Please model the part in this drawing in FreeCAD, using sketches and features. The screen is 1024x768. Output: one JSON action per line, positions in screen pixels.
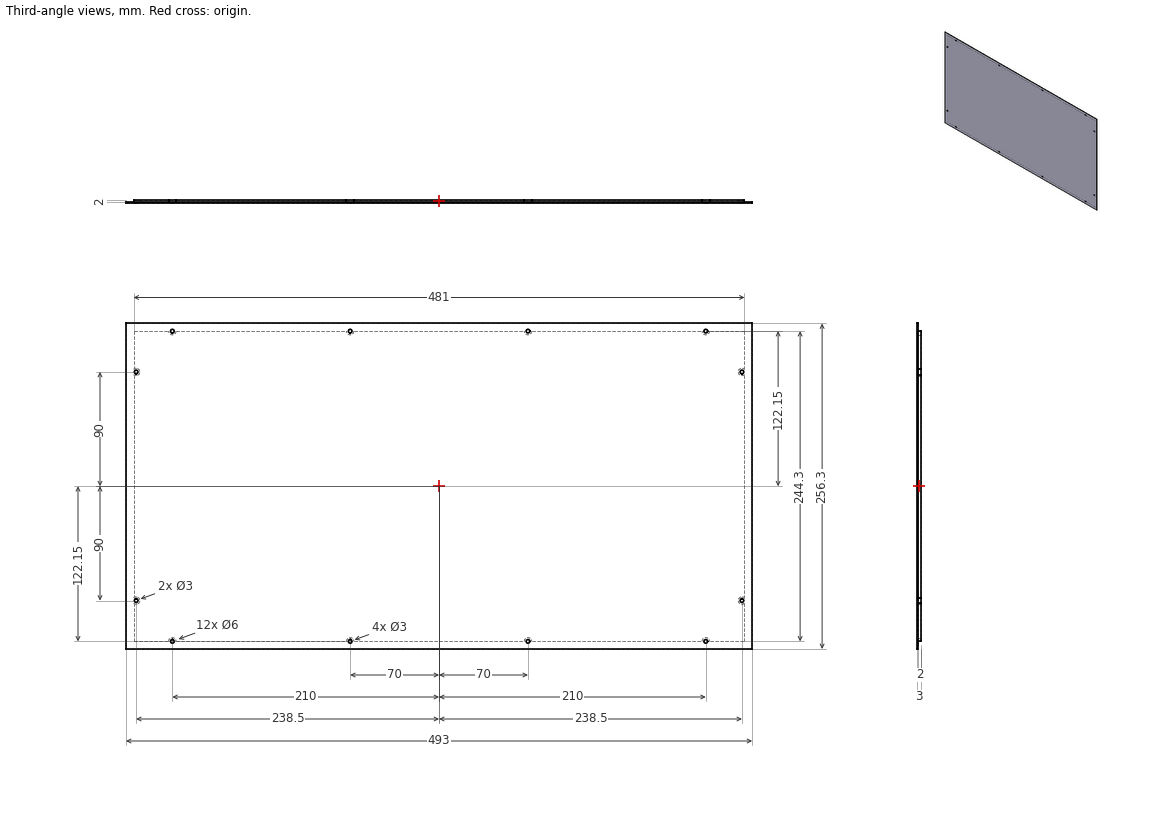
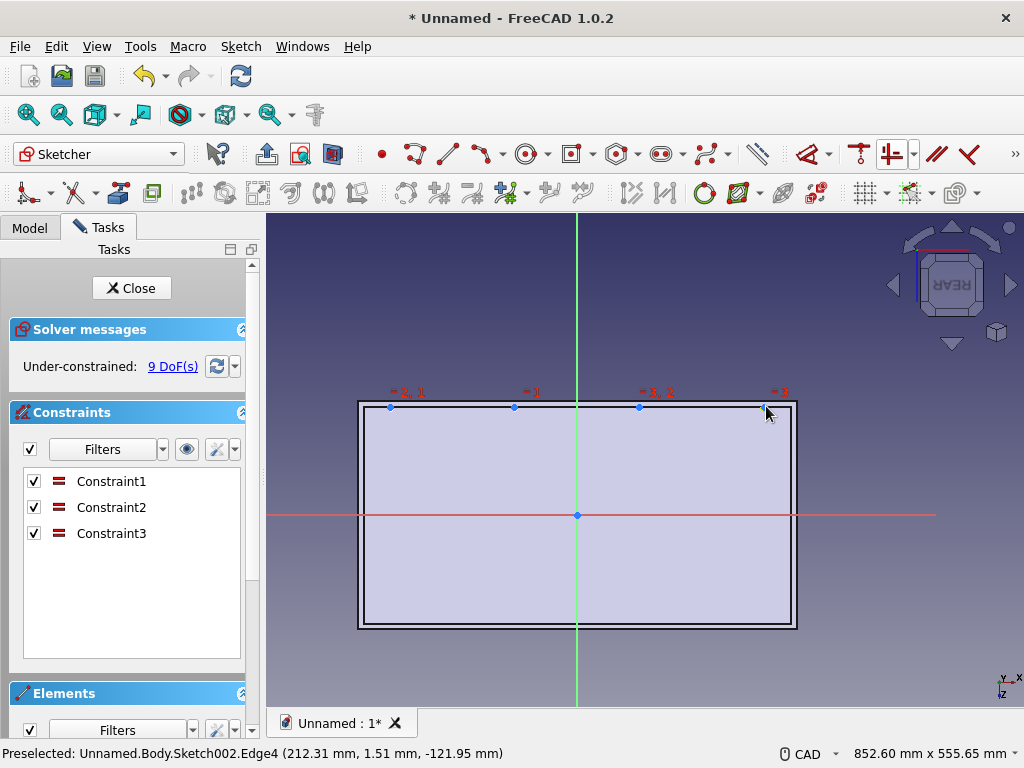
{"action": "left_click", "coordinate": [515, 408]}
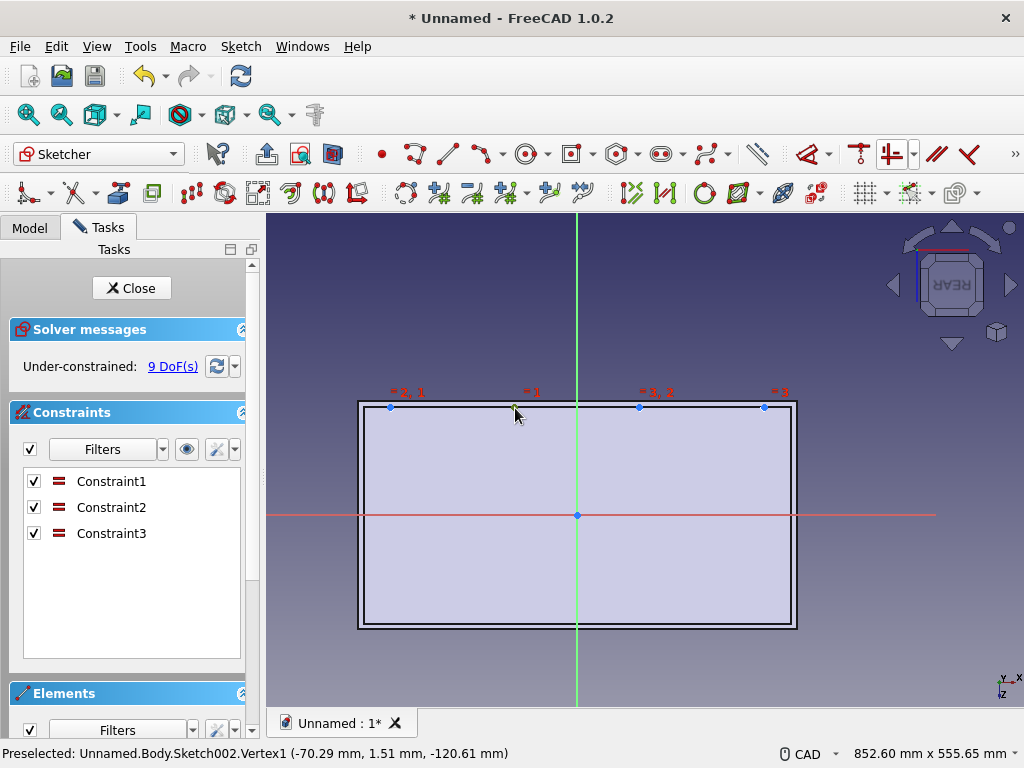
{"action": "left_click", "coordinate": [391, 408]}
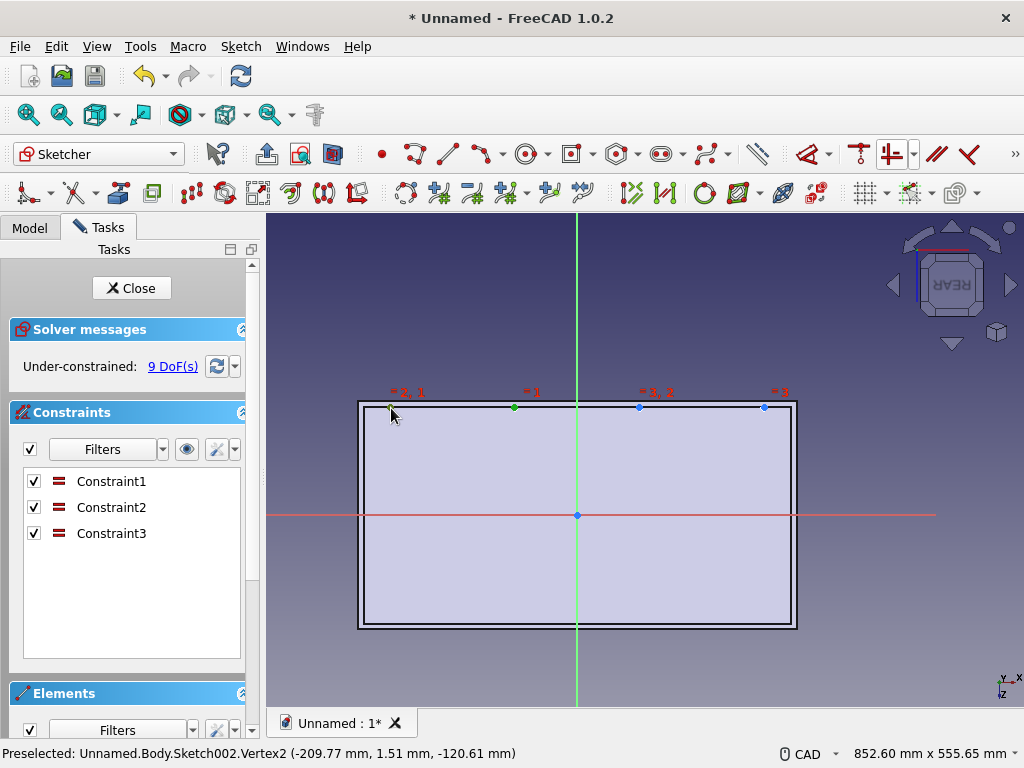
{"action": "left_click", "coordinate": [914, 154]}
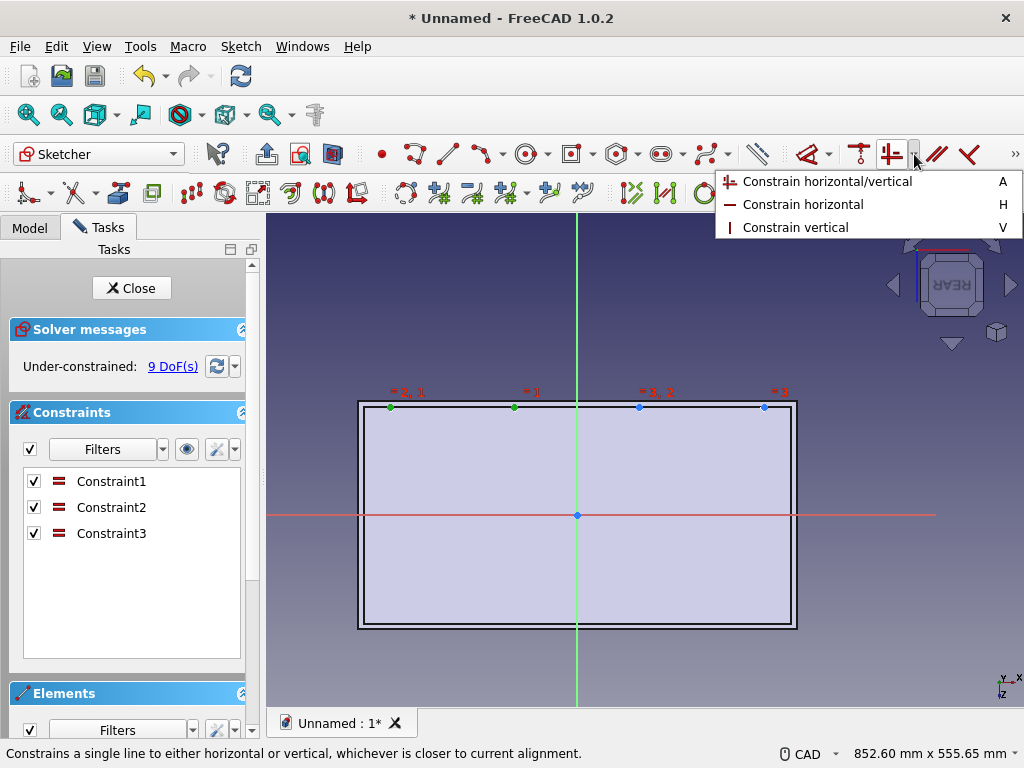
{"action": "left_click", "coordinate": [869, 204]}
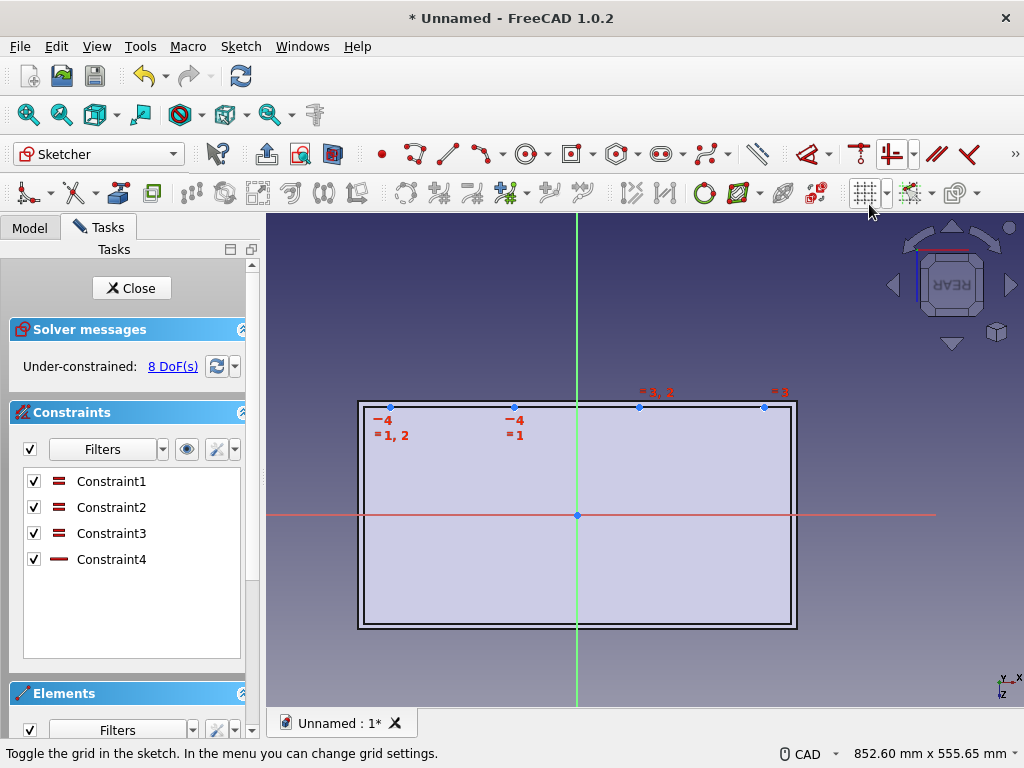
{"action": "left_click", "coordinate": [515, 408]}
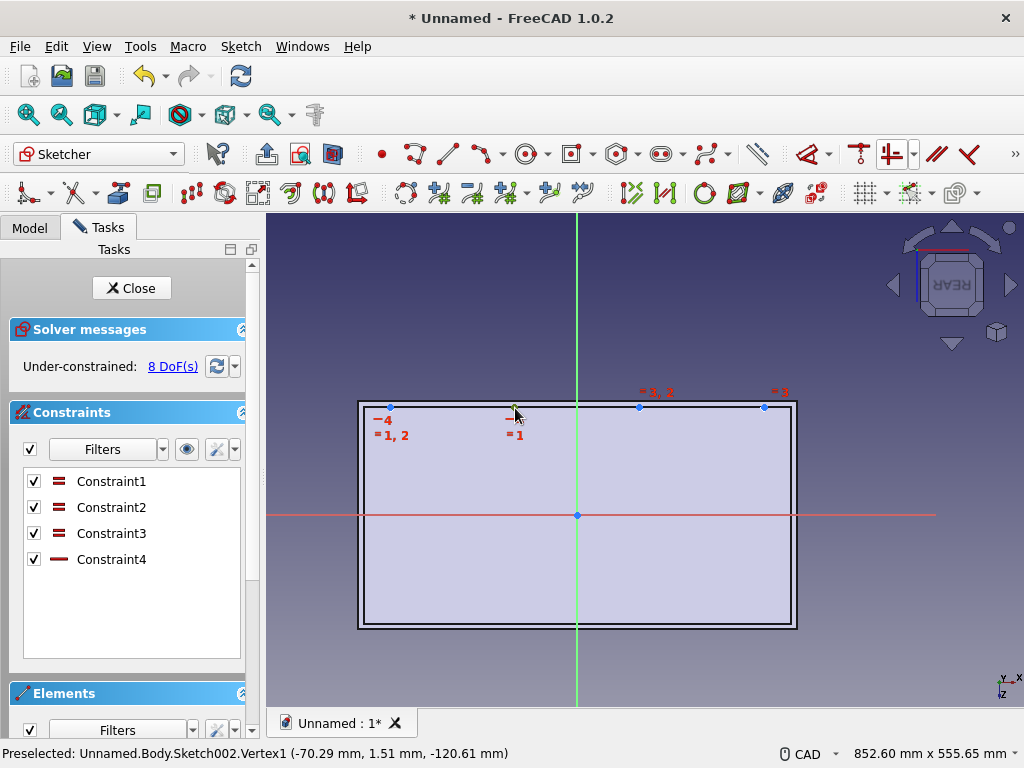
{"action": "left_click", "coordinate": [640, 408]}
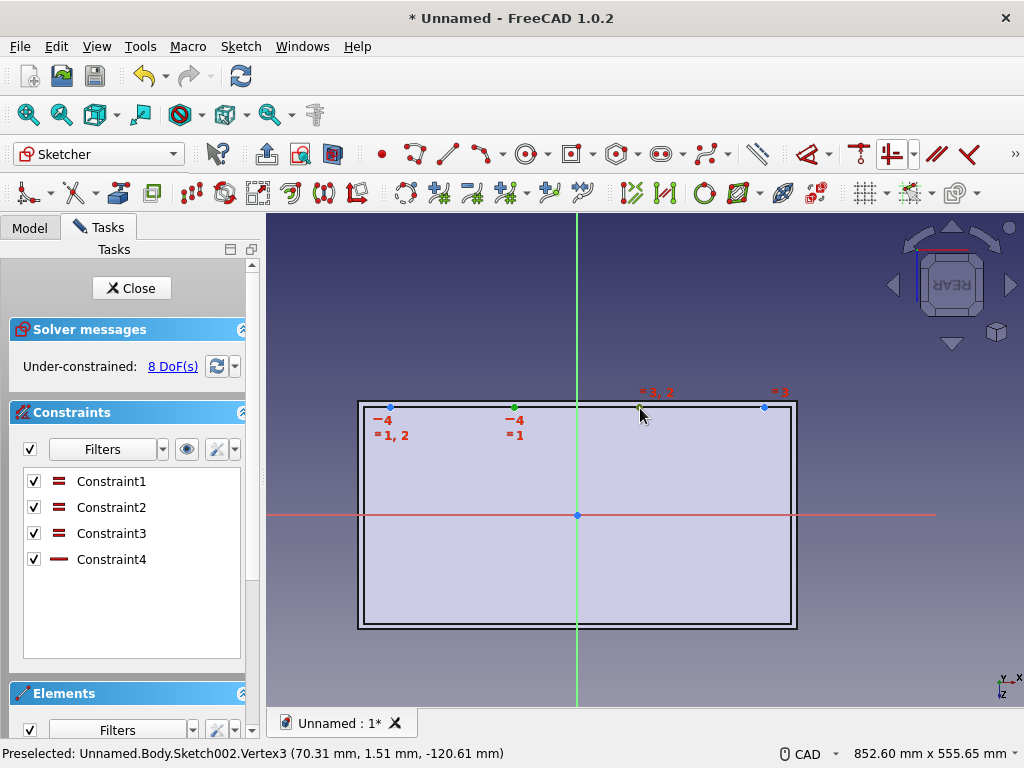
{"action": "left_click", "coordinate": [914, 154]}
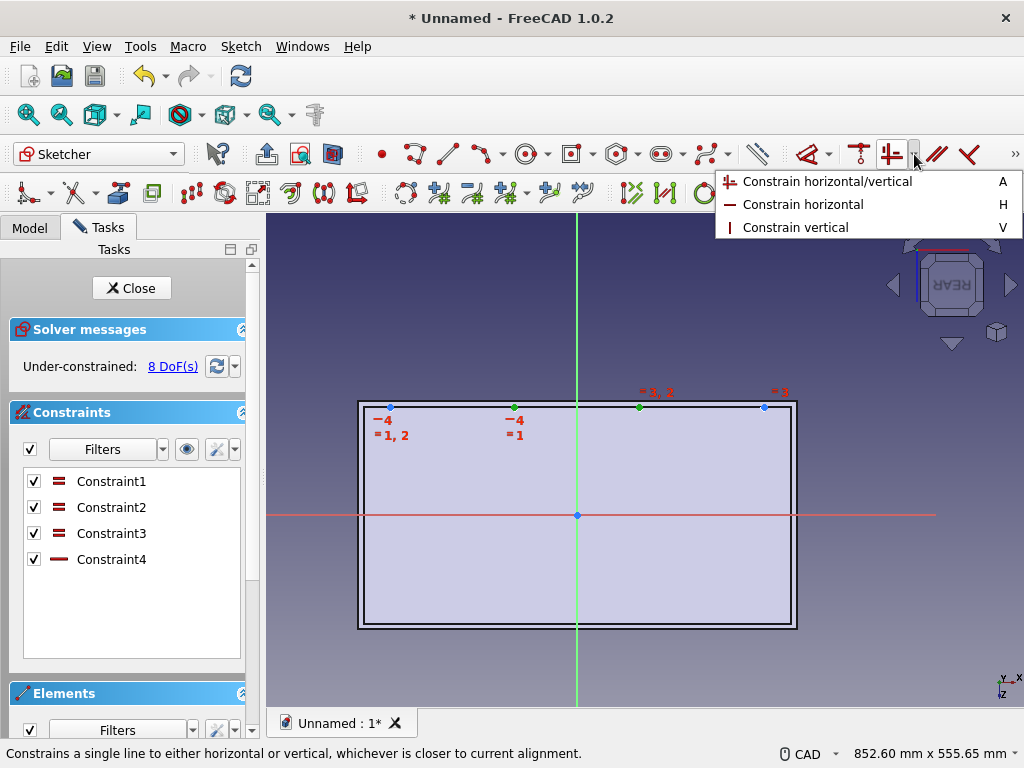
{"action": "left_click", "coordinate": [869, 204]}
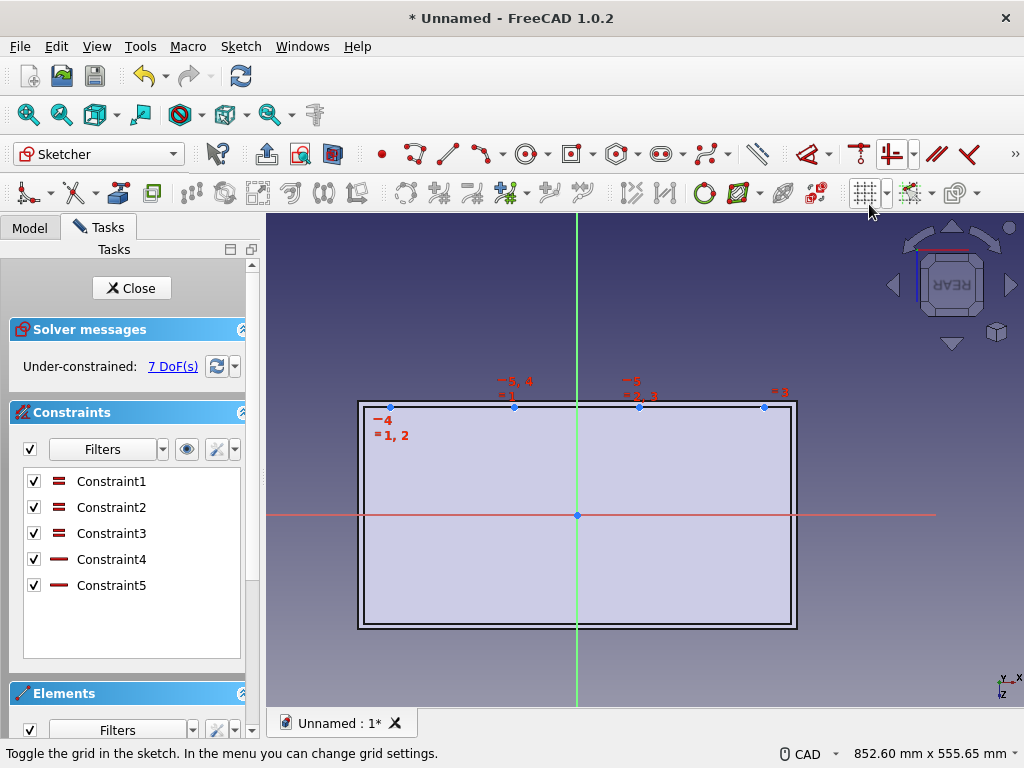
{"action": "left_click", "coordinate": [640, 408]}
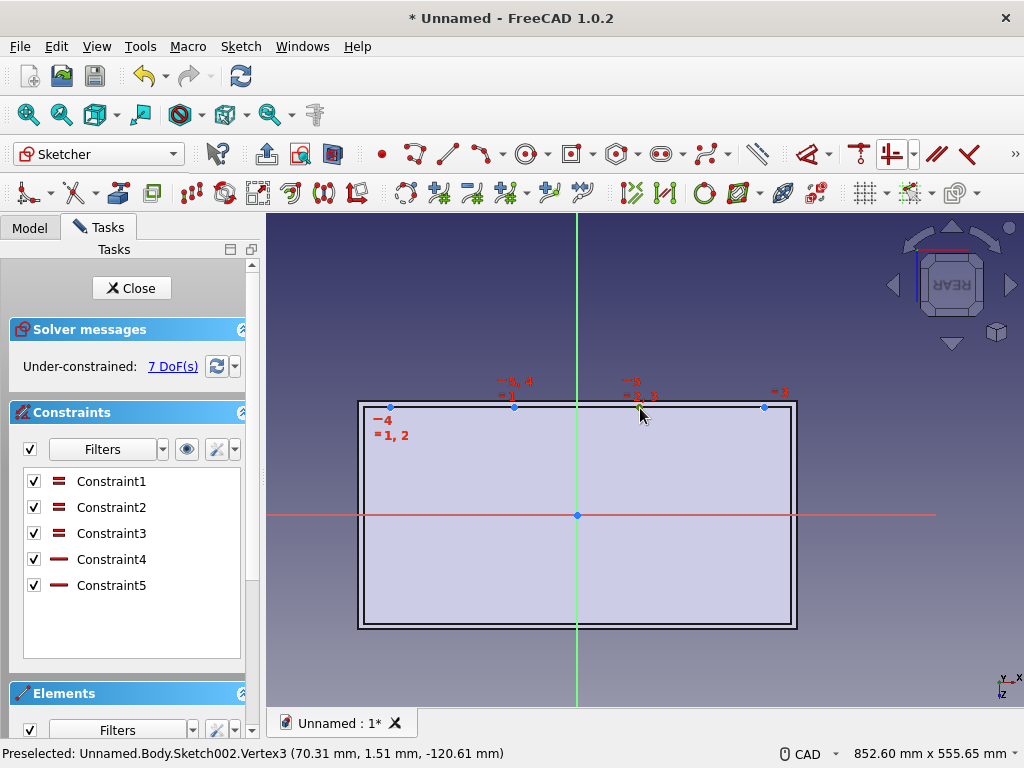
{"action": "left_click", "coordinate": [764, 408]}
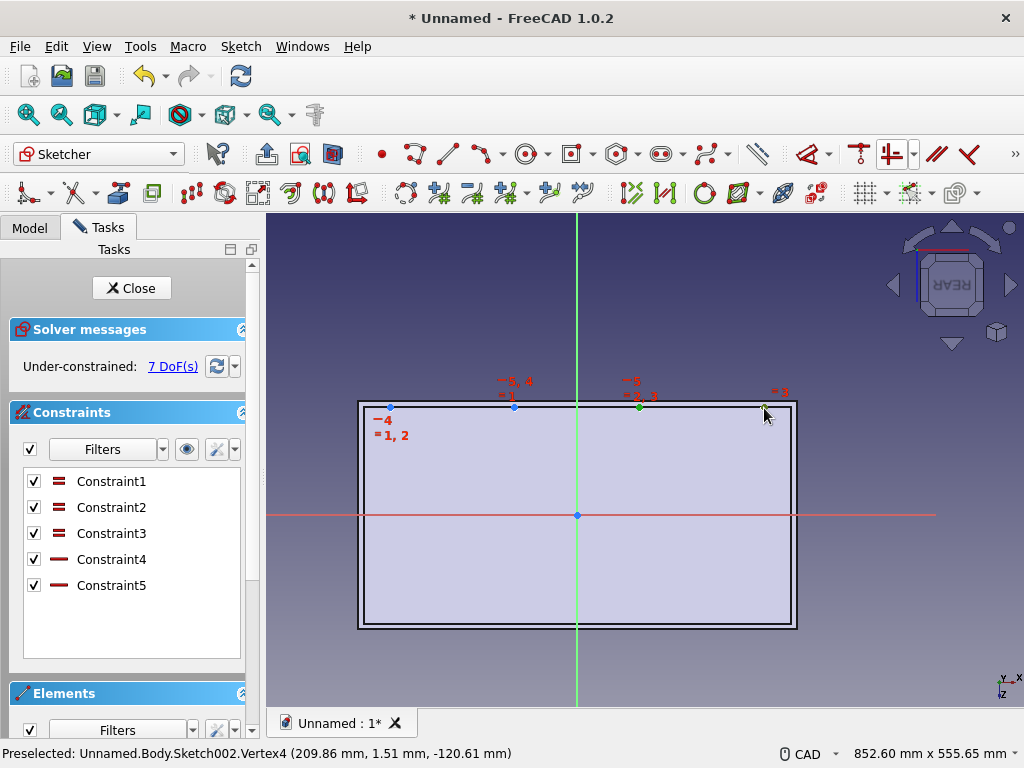
{"action": "left_click", "coordinate": [914, 154]}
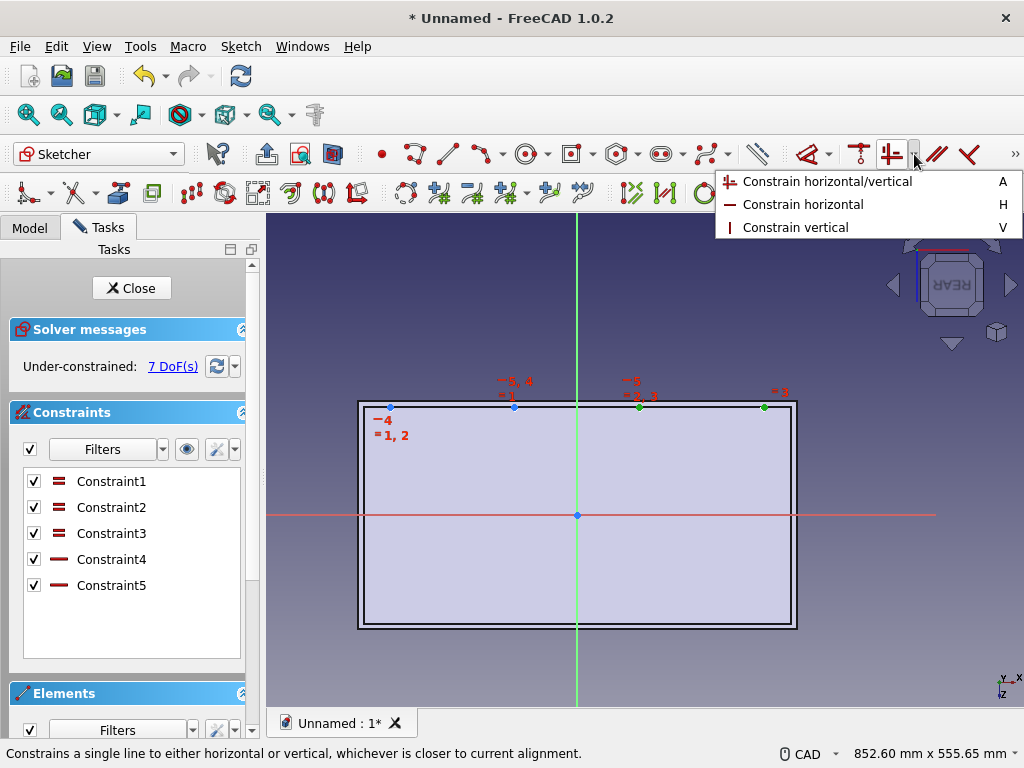
{"action": "left_click", "coordinate": [869, 204]}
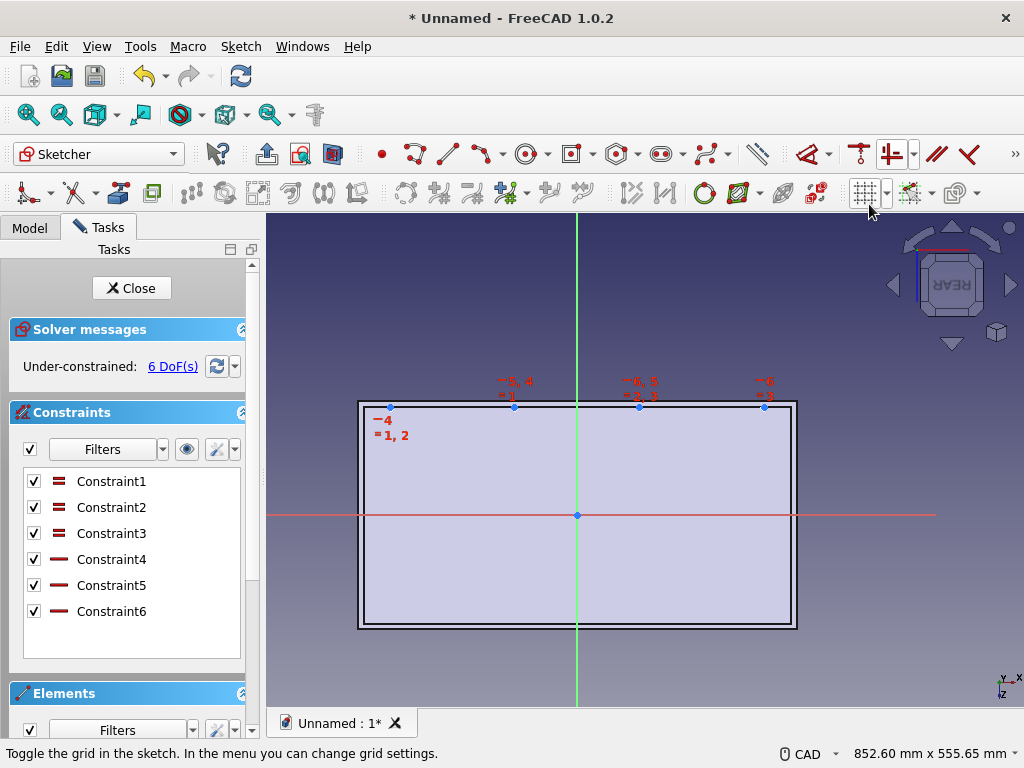
{"action": "left_click", "coordinate": [806, 154]}